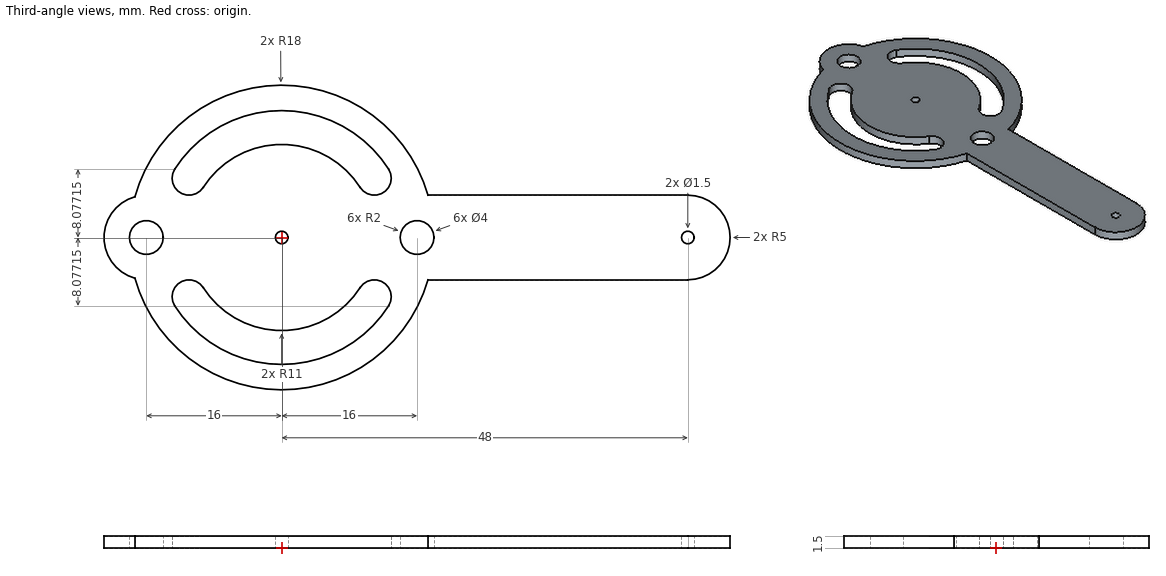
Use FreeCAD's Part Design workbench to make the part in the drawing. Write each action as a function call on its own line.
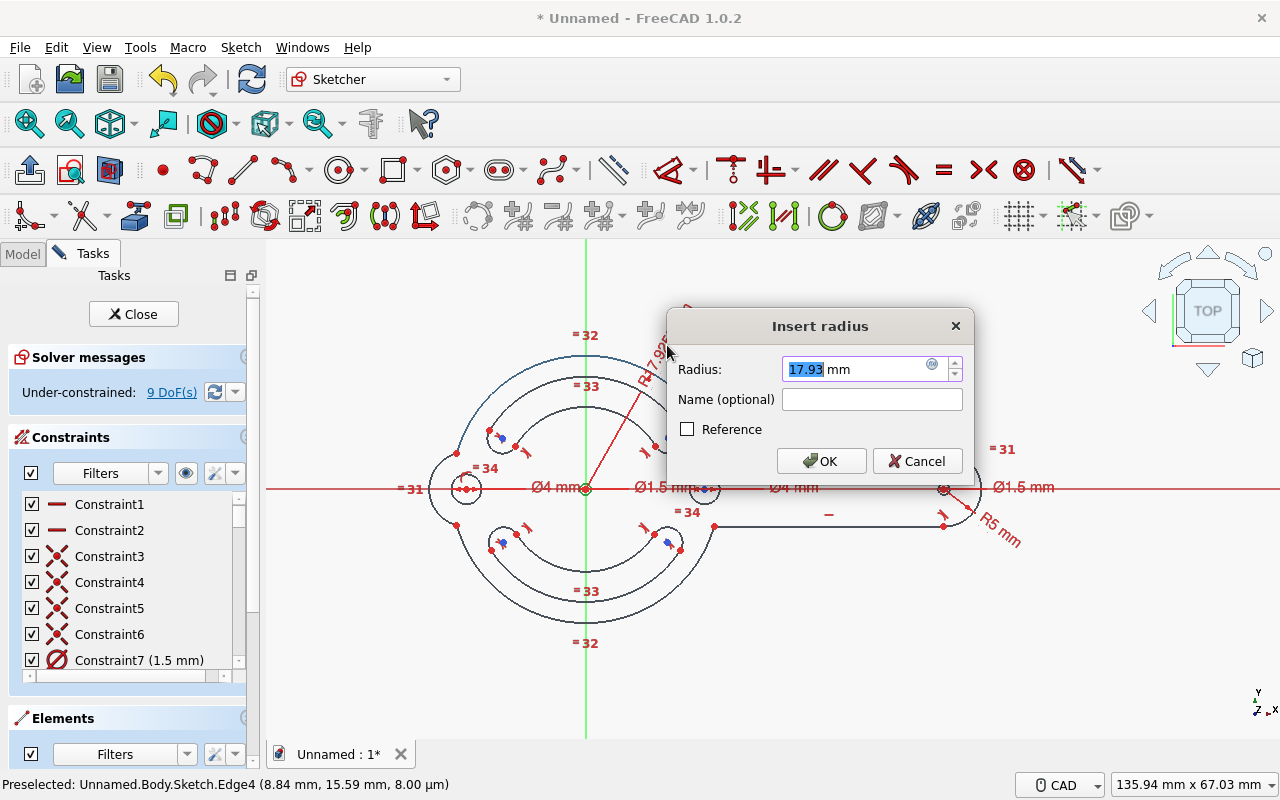
text(18)
key(Return)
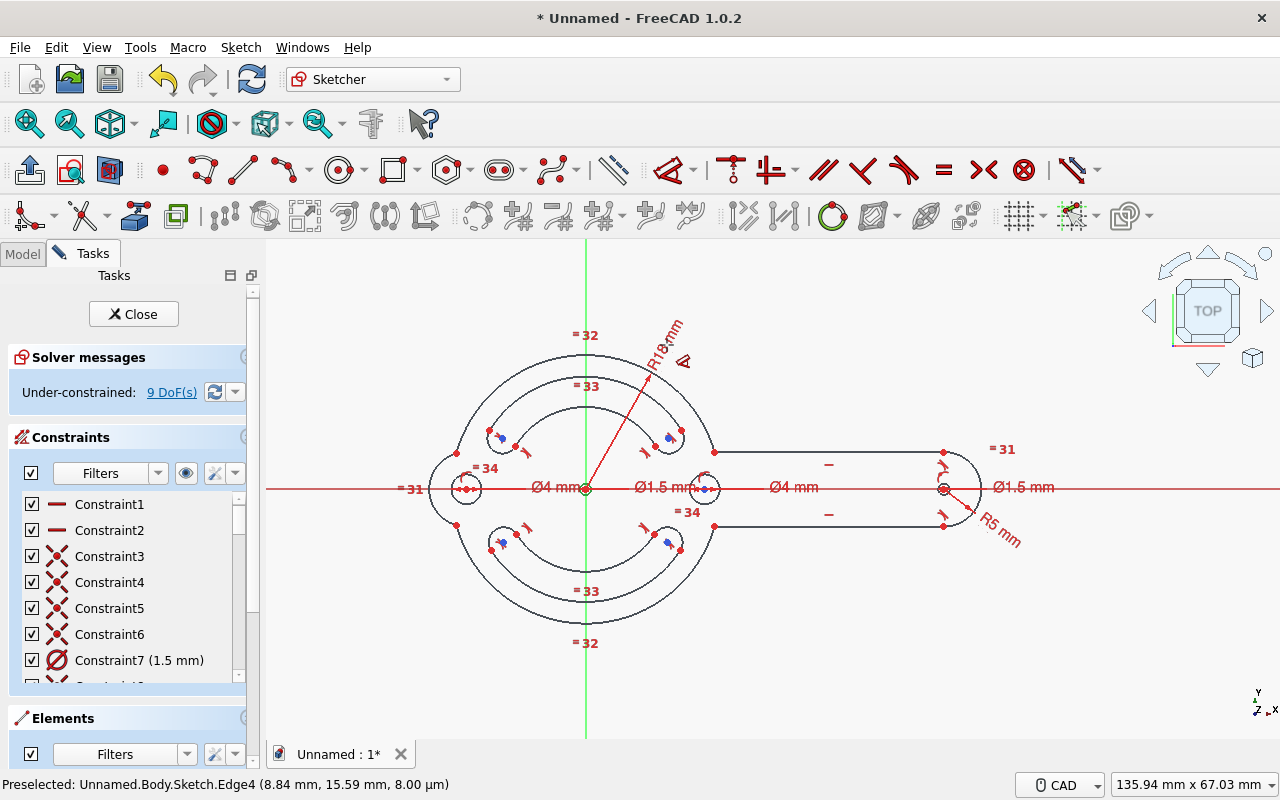
click(554, 565)
click(523, 639)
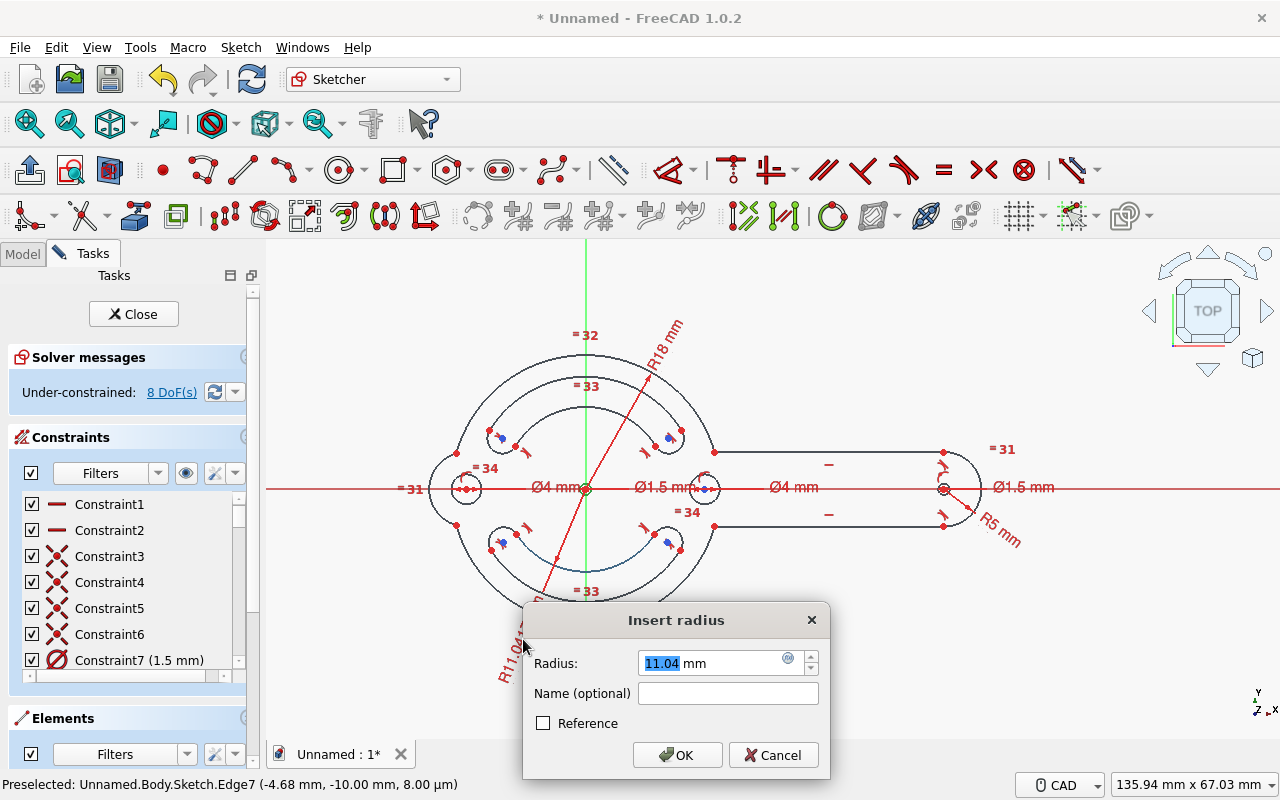
text(11)
key(Return)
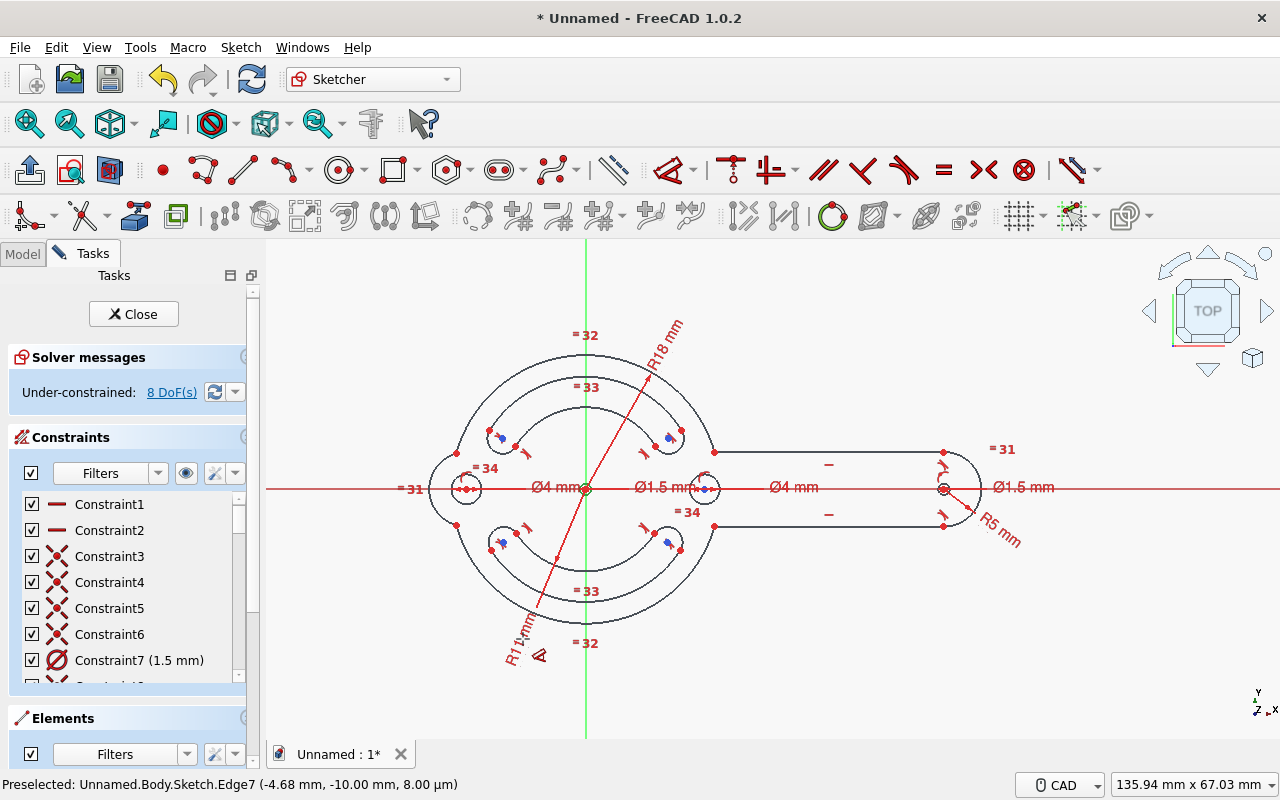
scroll(682, 537, up, 5)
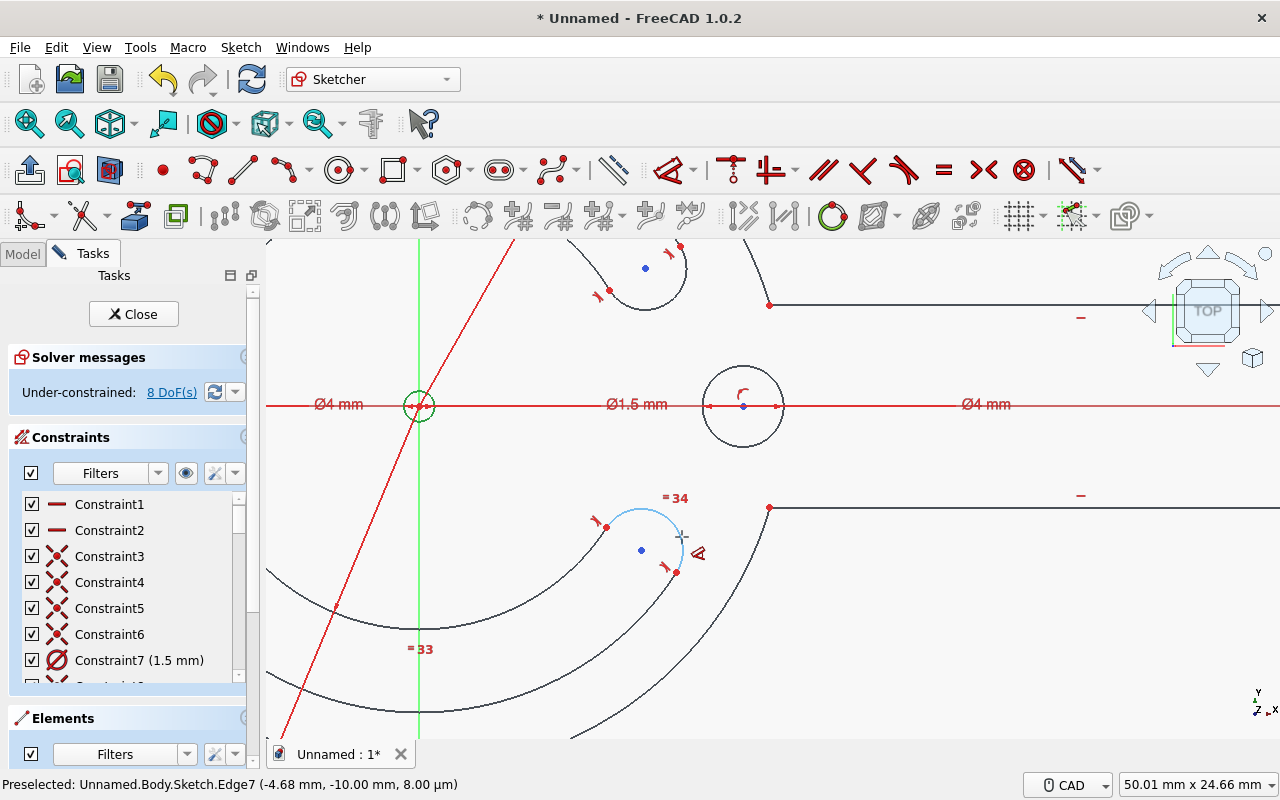
click(680, 535)
click(710, 523)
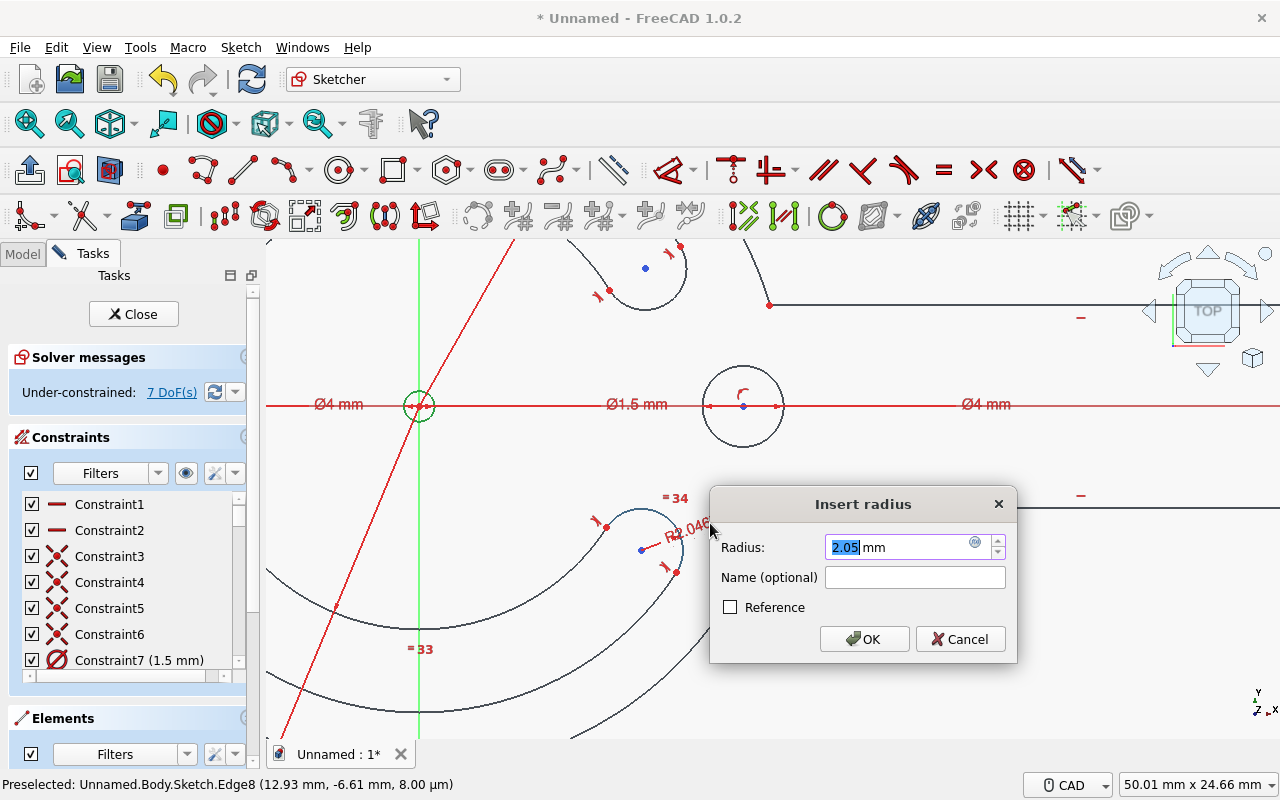
text(2)
key(Return)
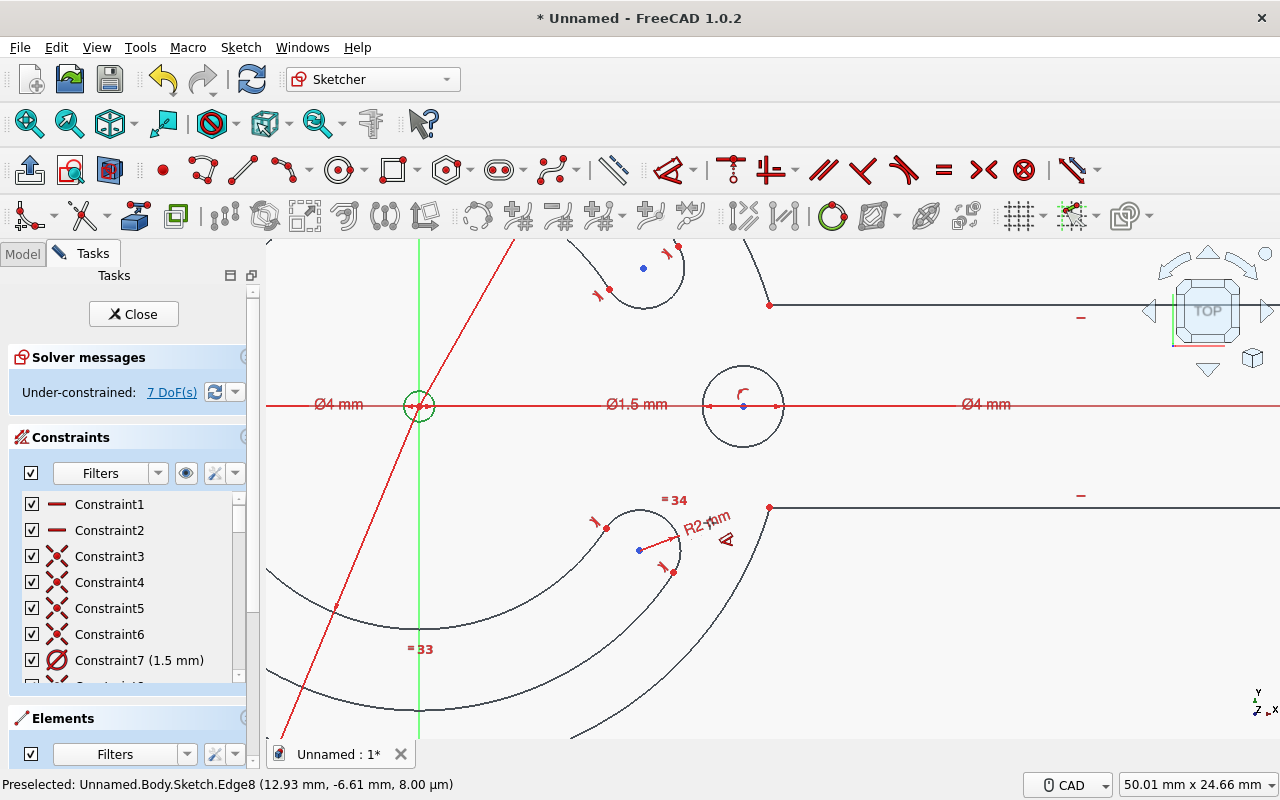
scroll(682, 537, down, 5)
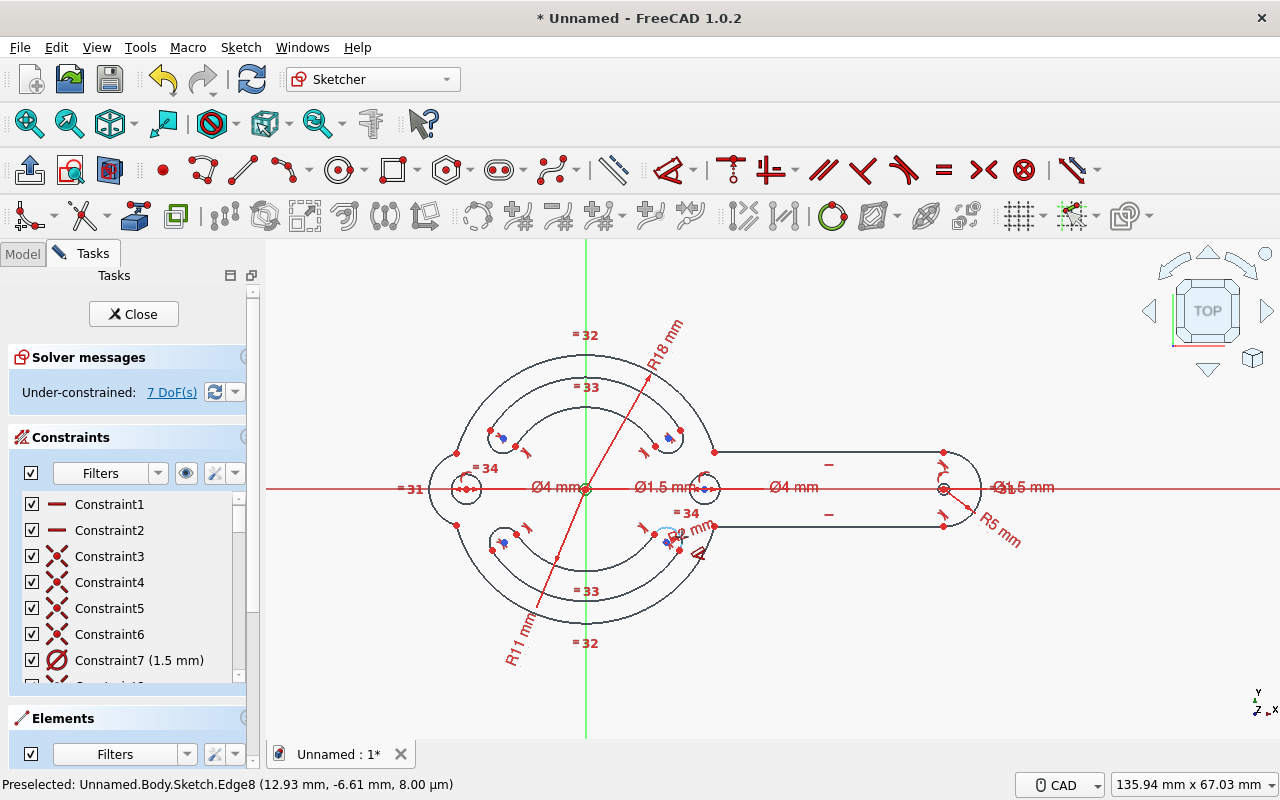
click(944, 489)
click(639, 455)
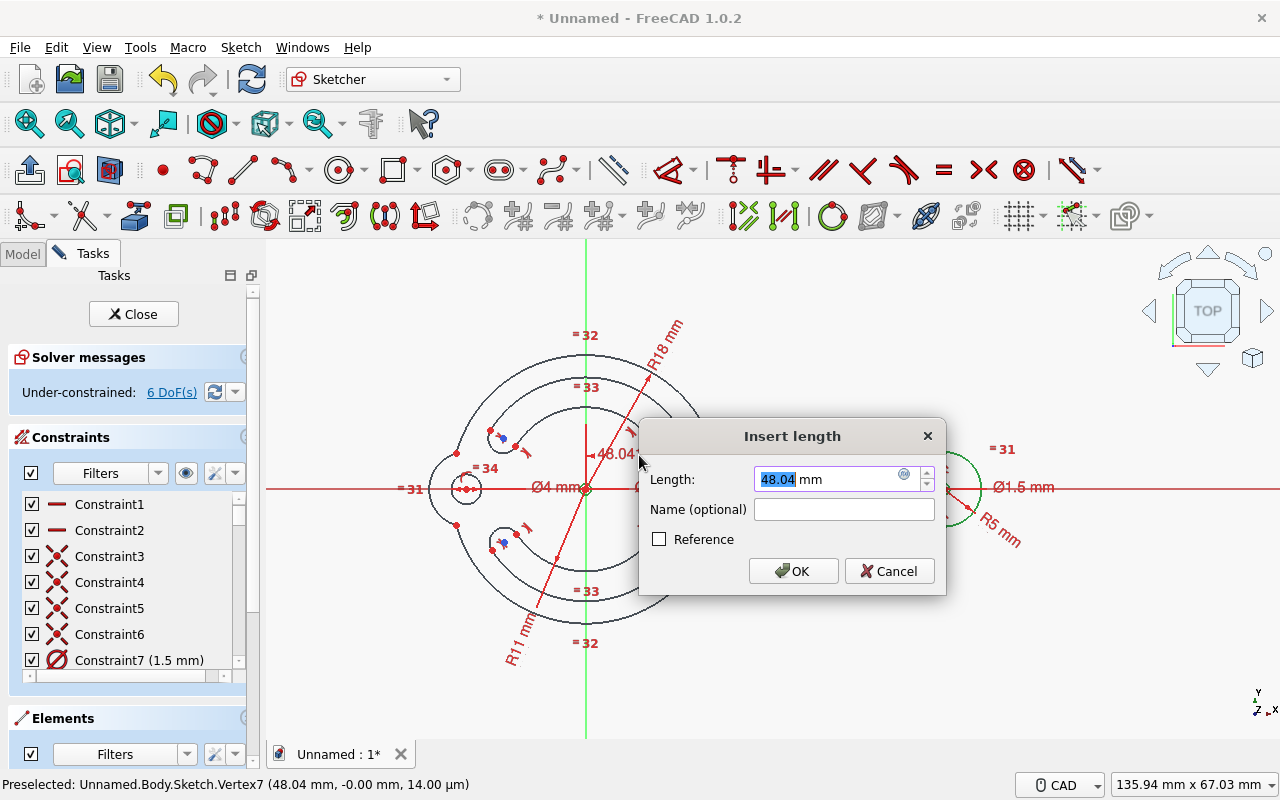
text(48)
key(Return)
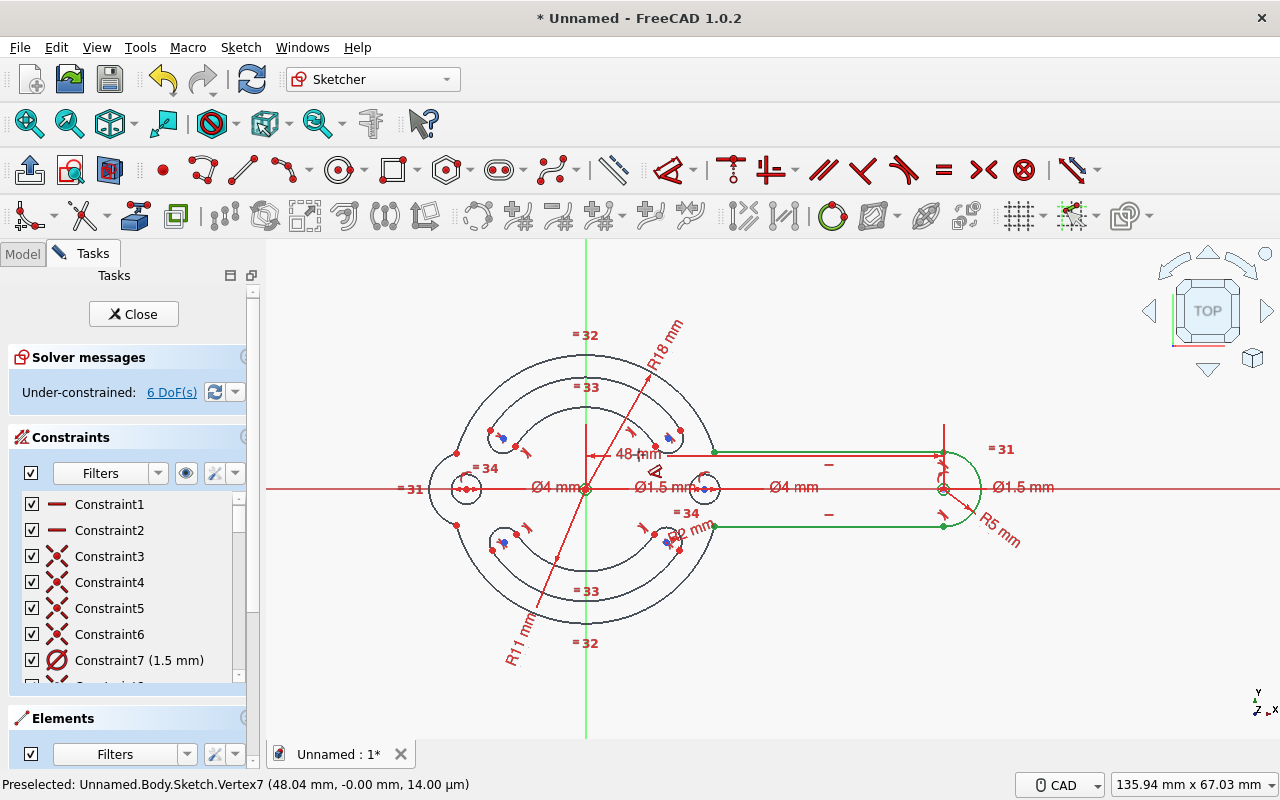
click(705, 489)
click(618, 523)